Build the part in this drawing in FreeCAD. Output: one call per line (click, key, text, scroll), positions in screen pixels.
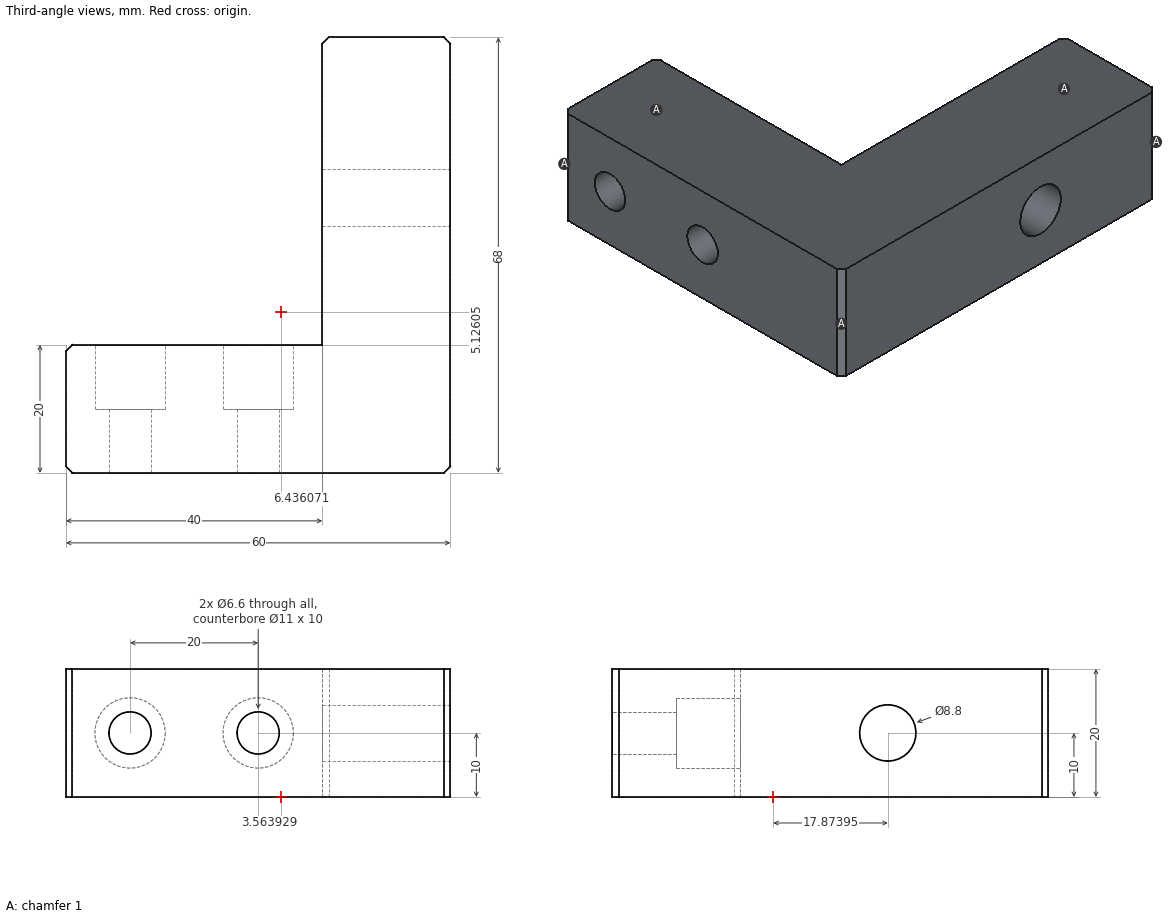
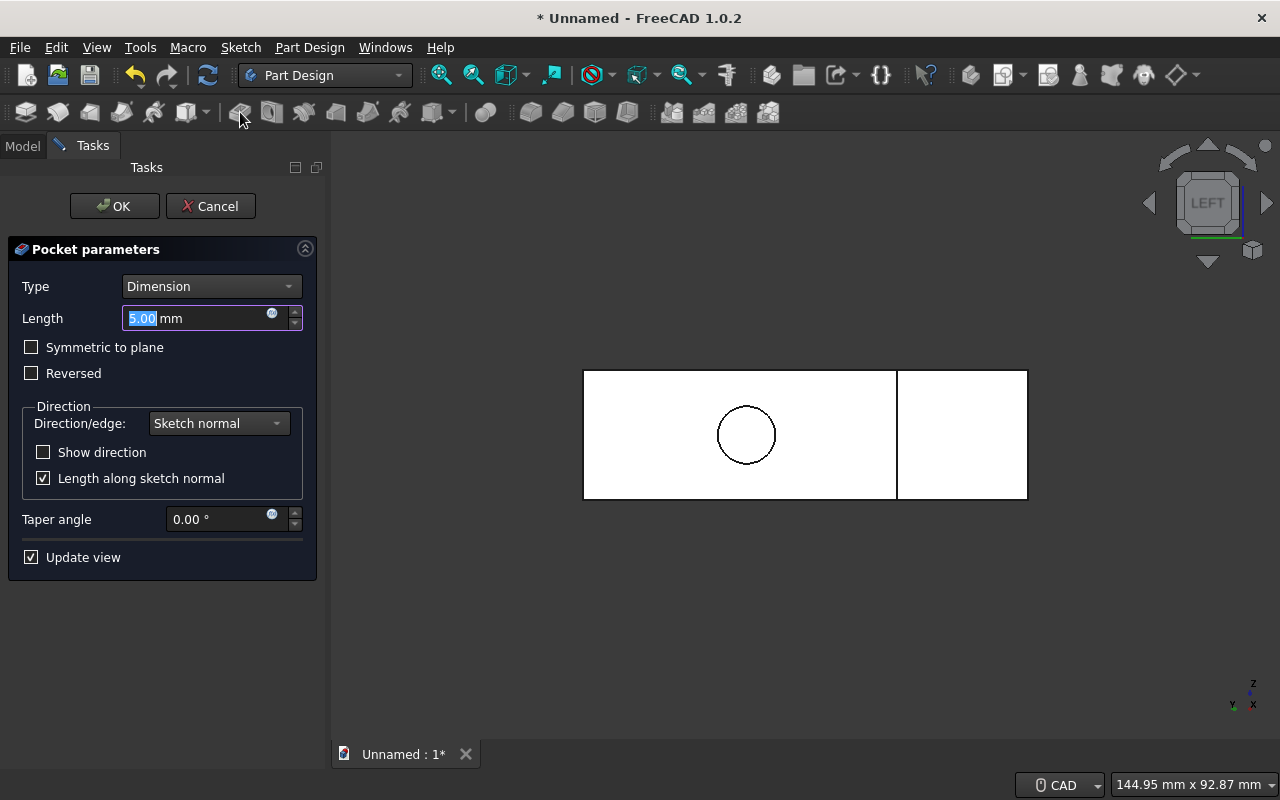
click(212, 286)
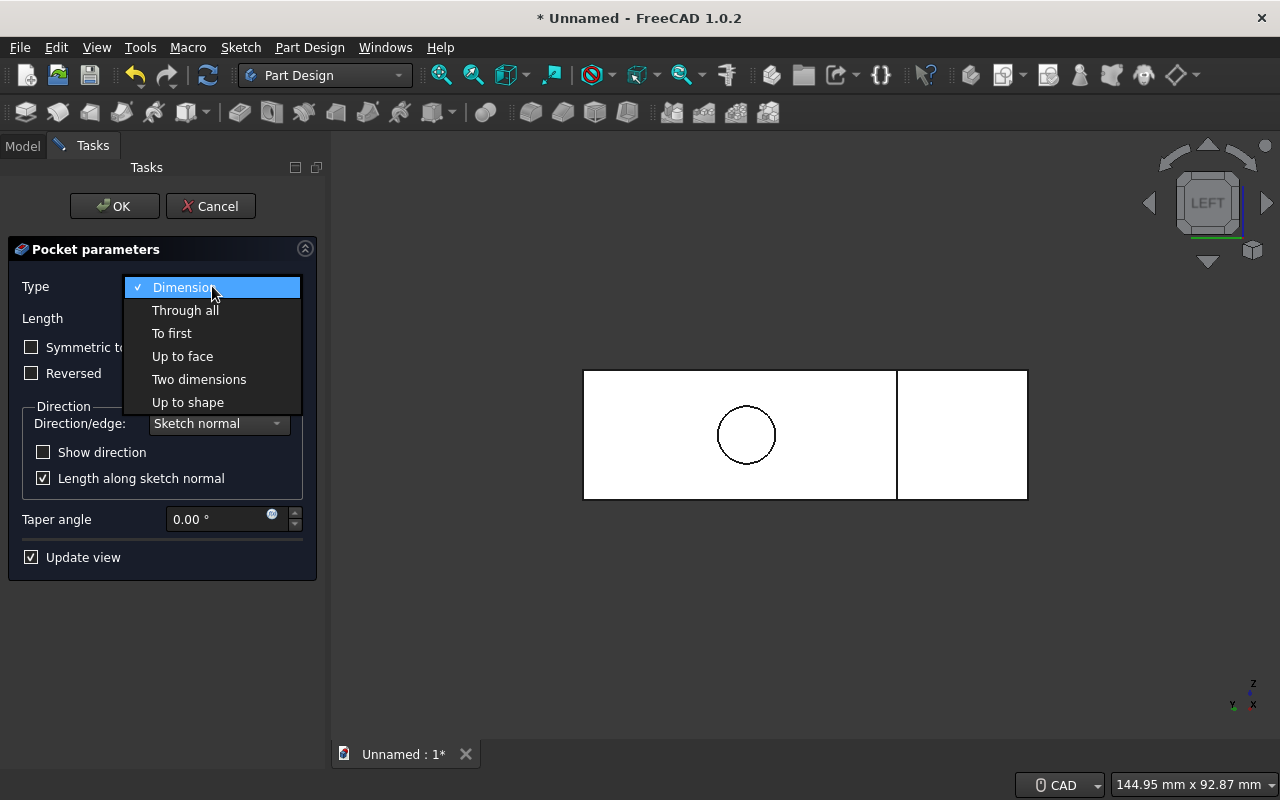
click(212, 310)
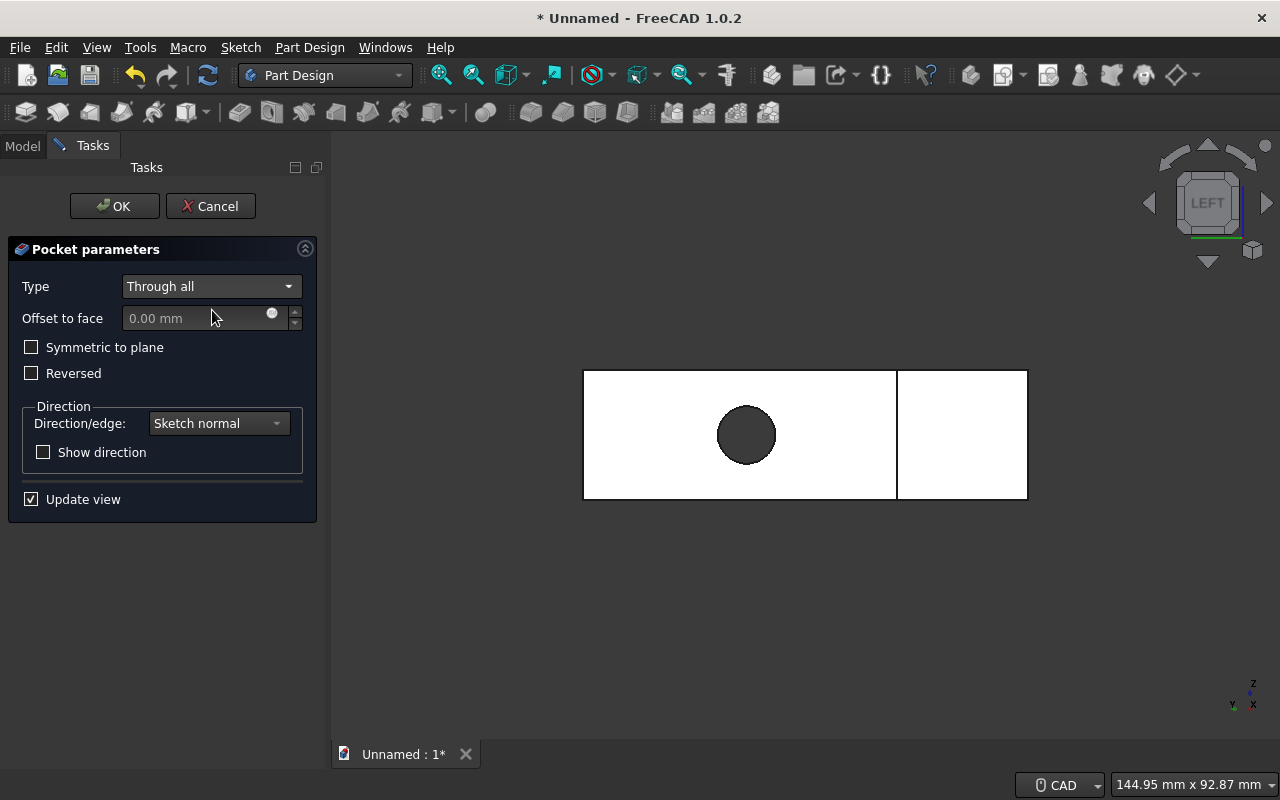
click(115, 206)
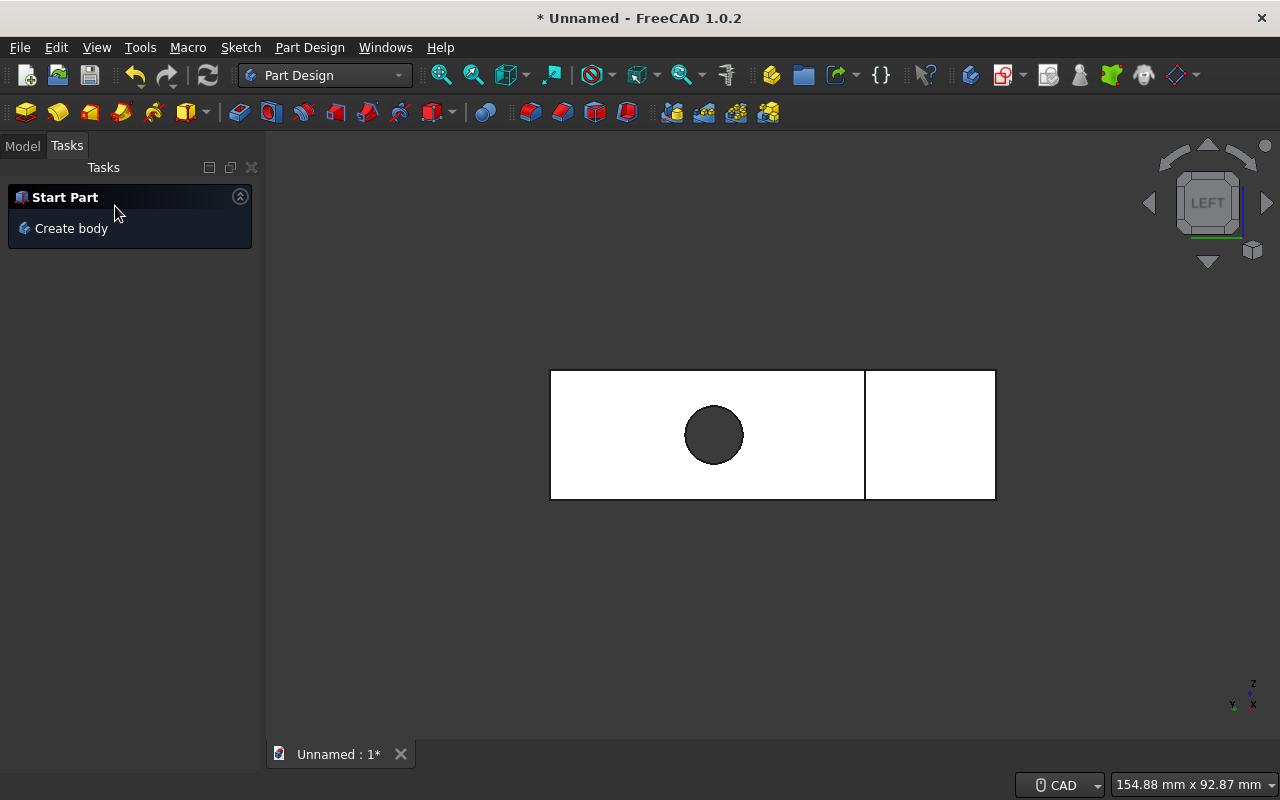
key(v)
key(f)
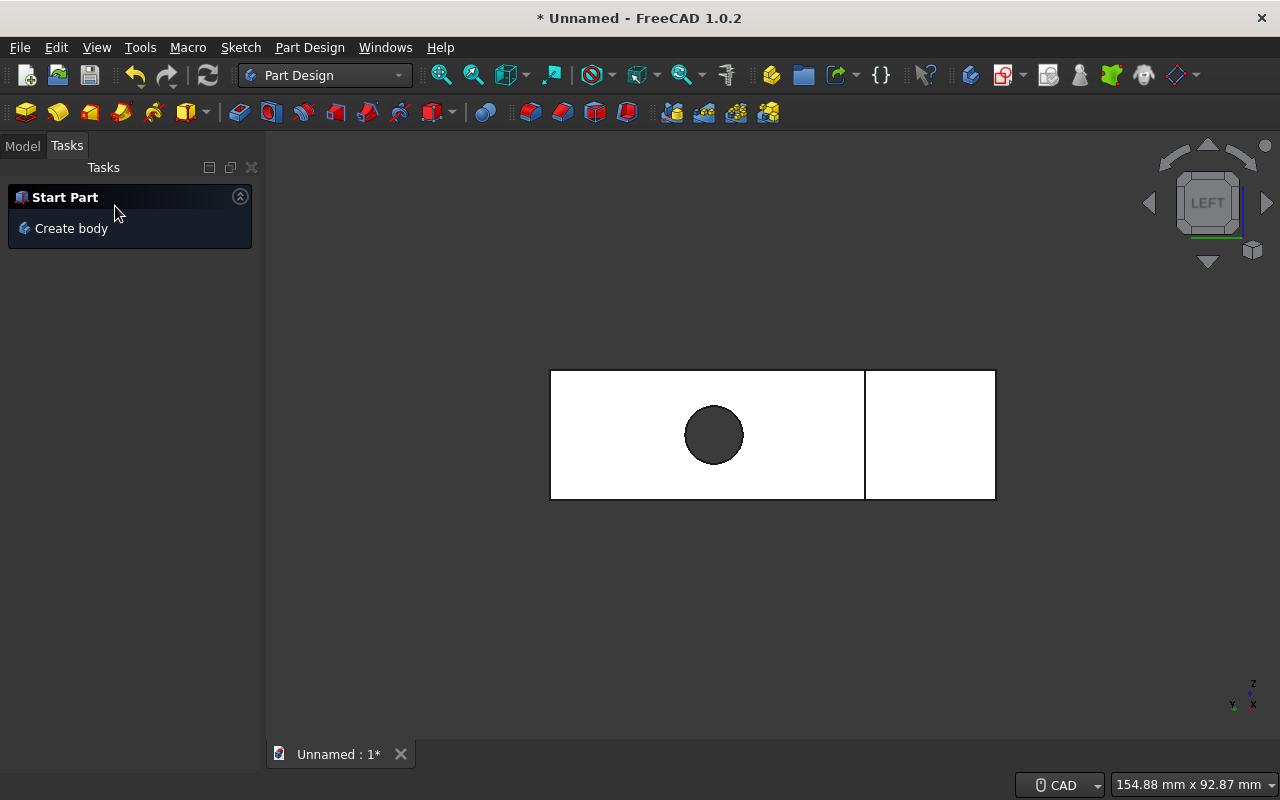
key(4)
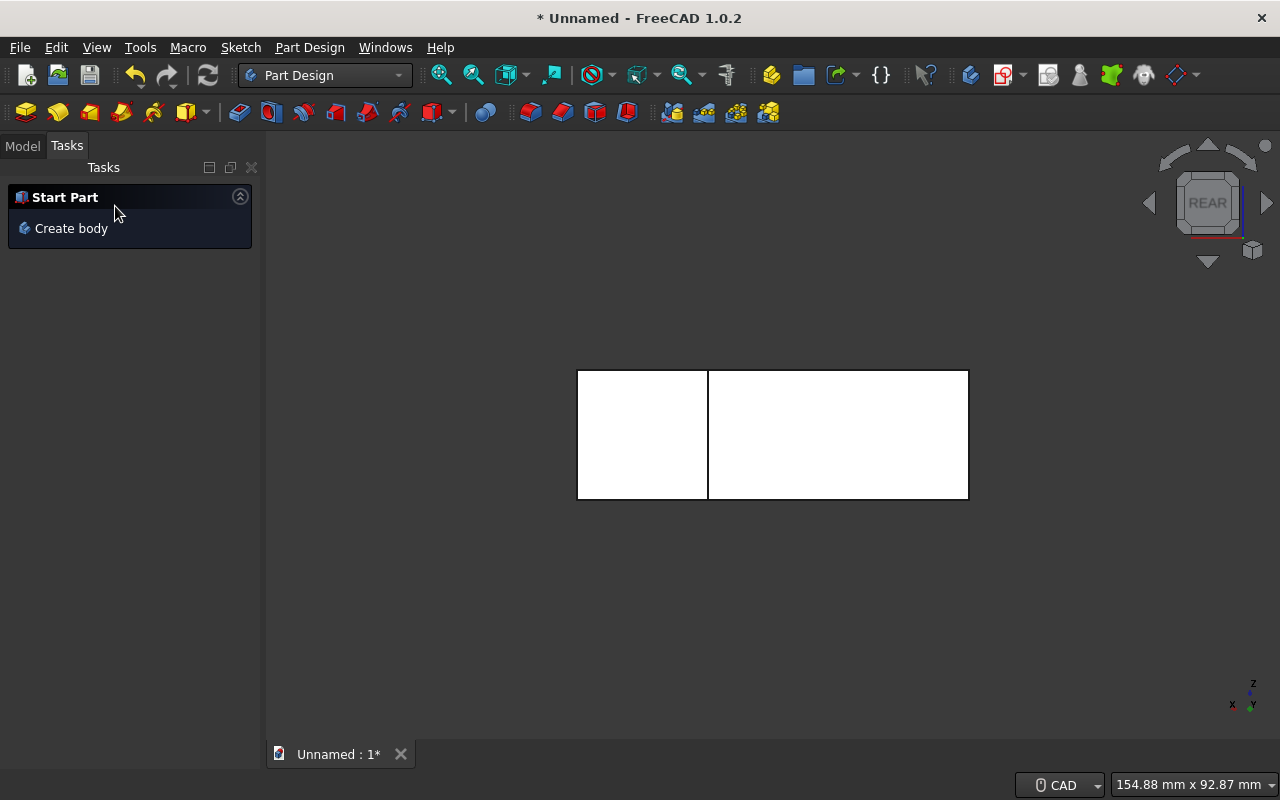
click(442, 76)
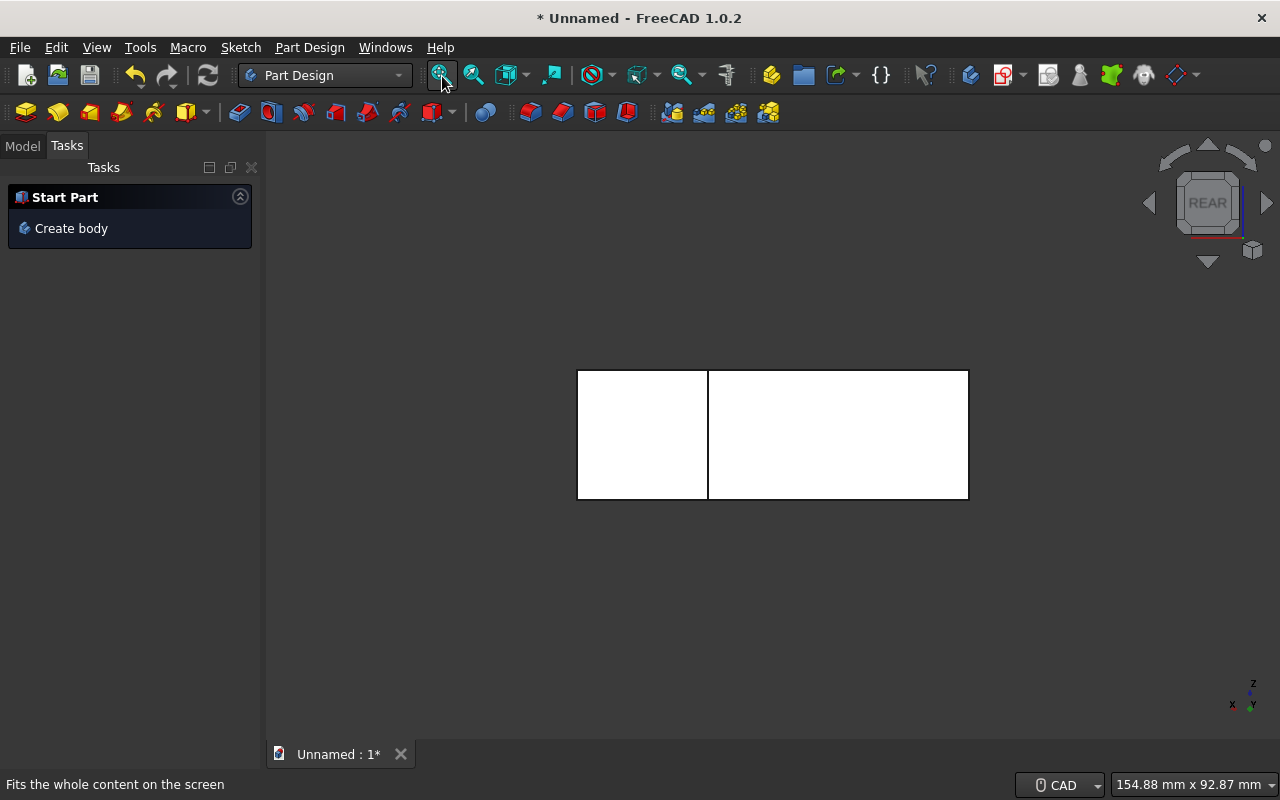
click(801, 434)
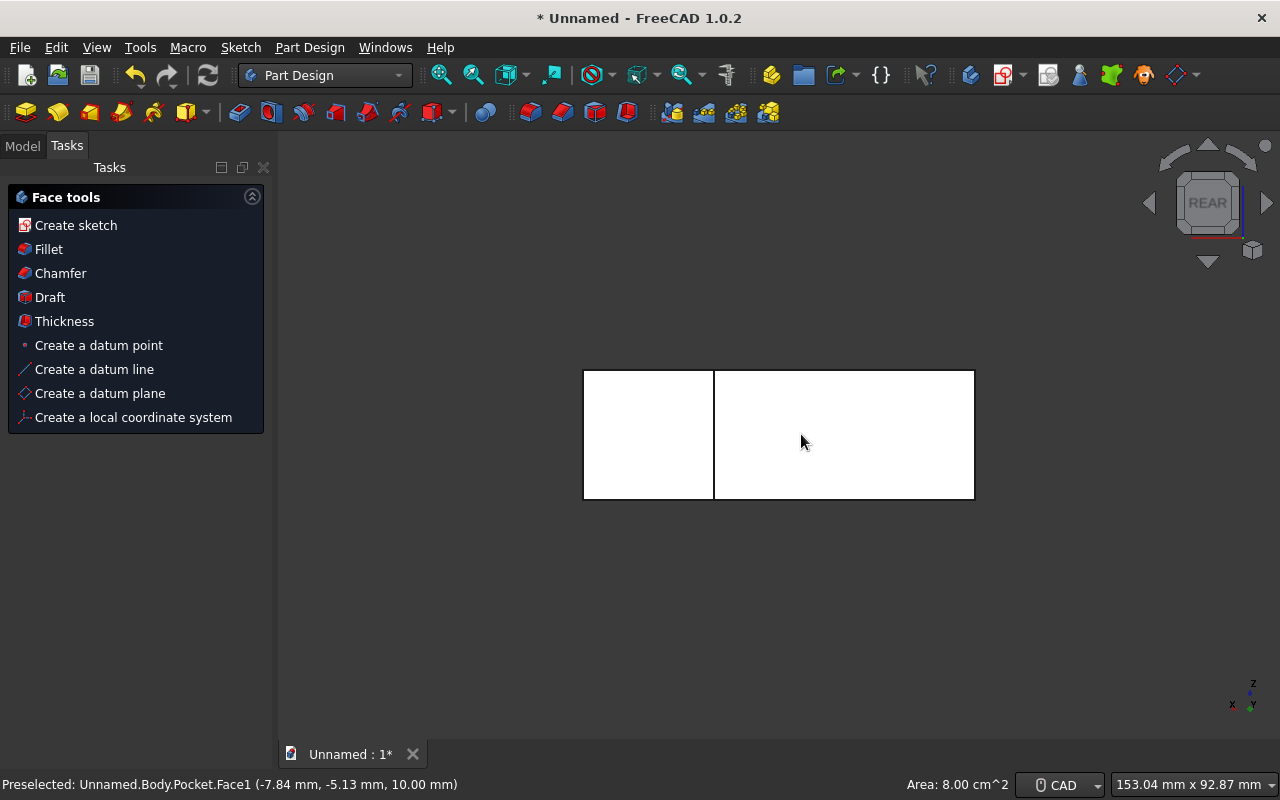
click(1004, 76)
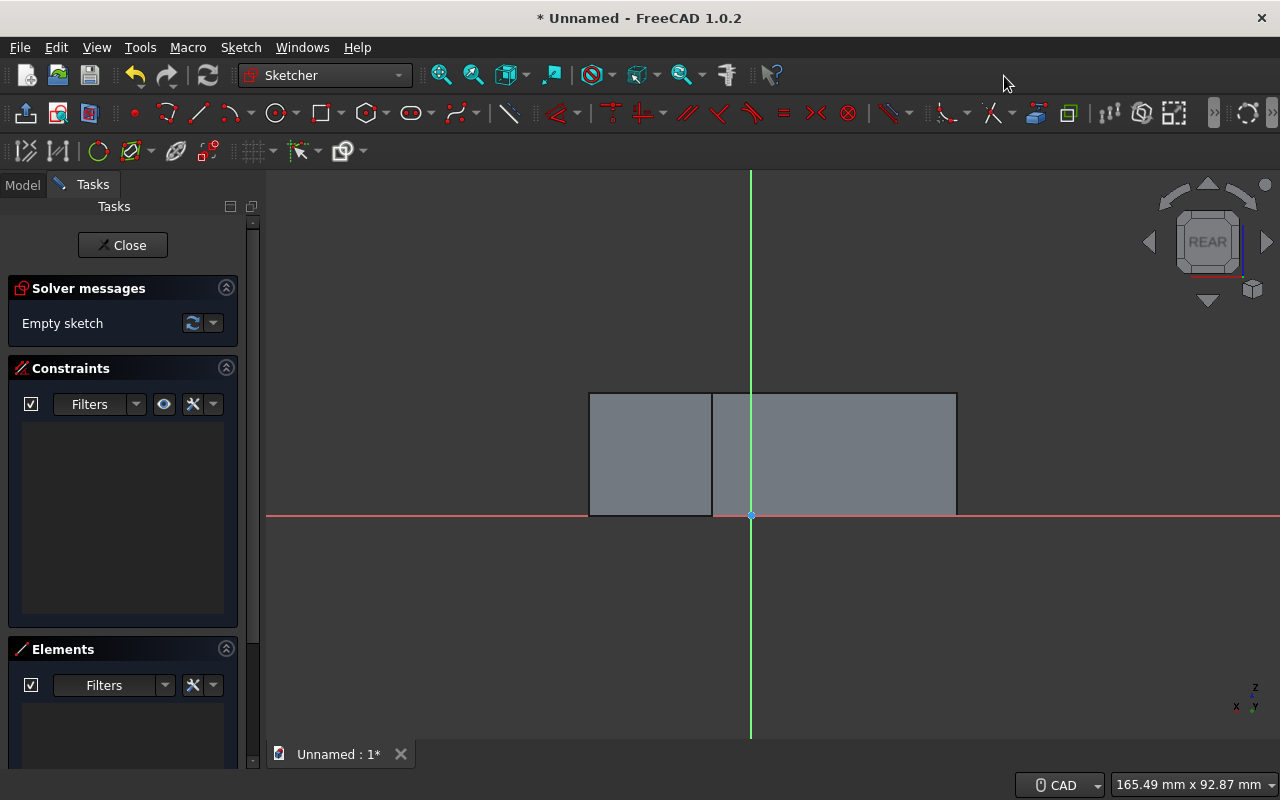
click(90, 114)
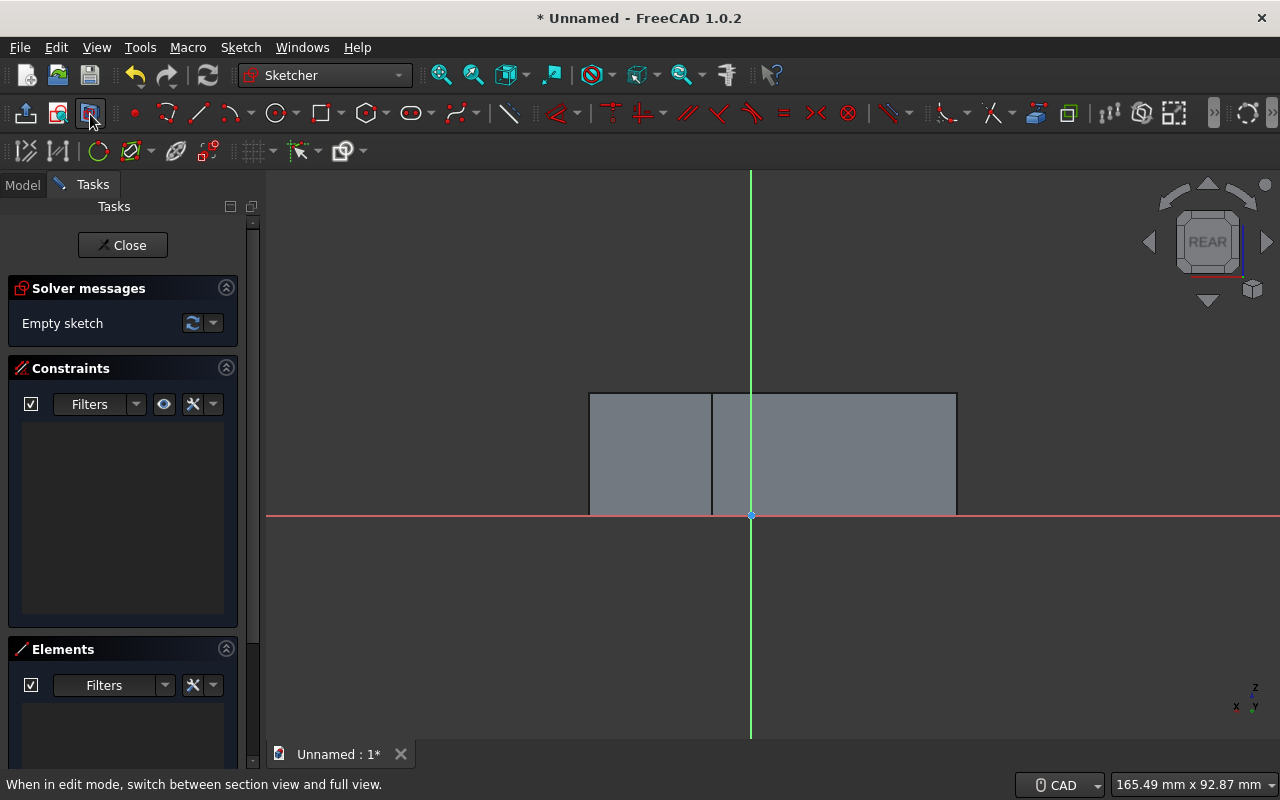
scroll(889, 484, up, 6)